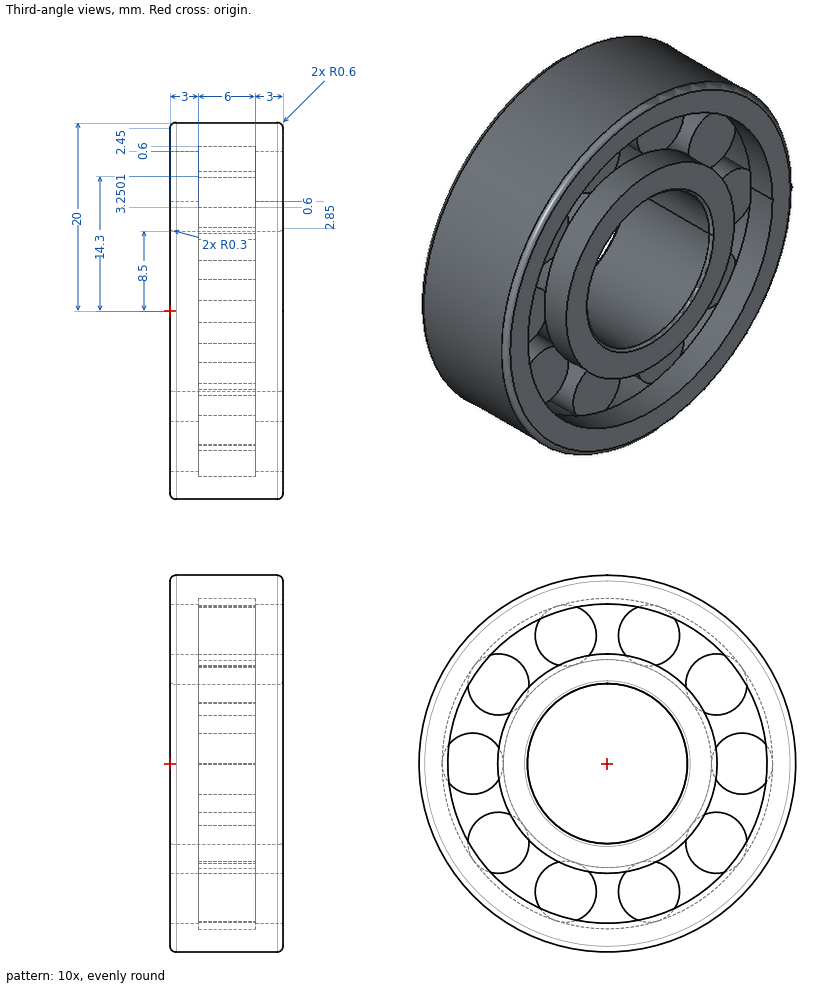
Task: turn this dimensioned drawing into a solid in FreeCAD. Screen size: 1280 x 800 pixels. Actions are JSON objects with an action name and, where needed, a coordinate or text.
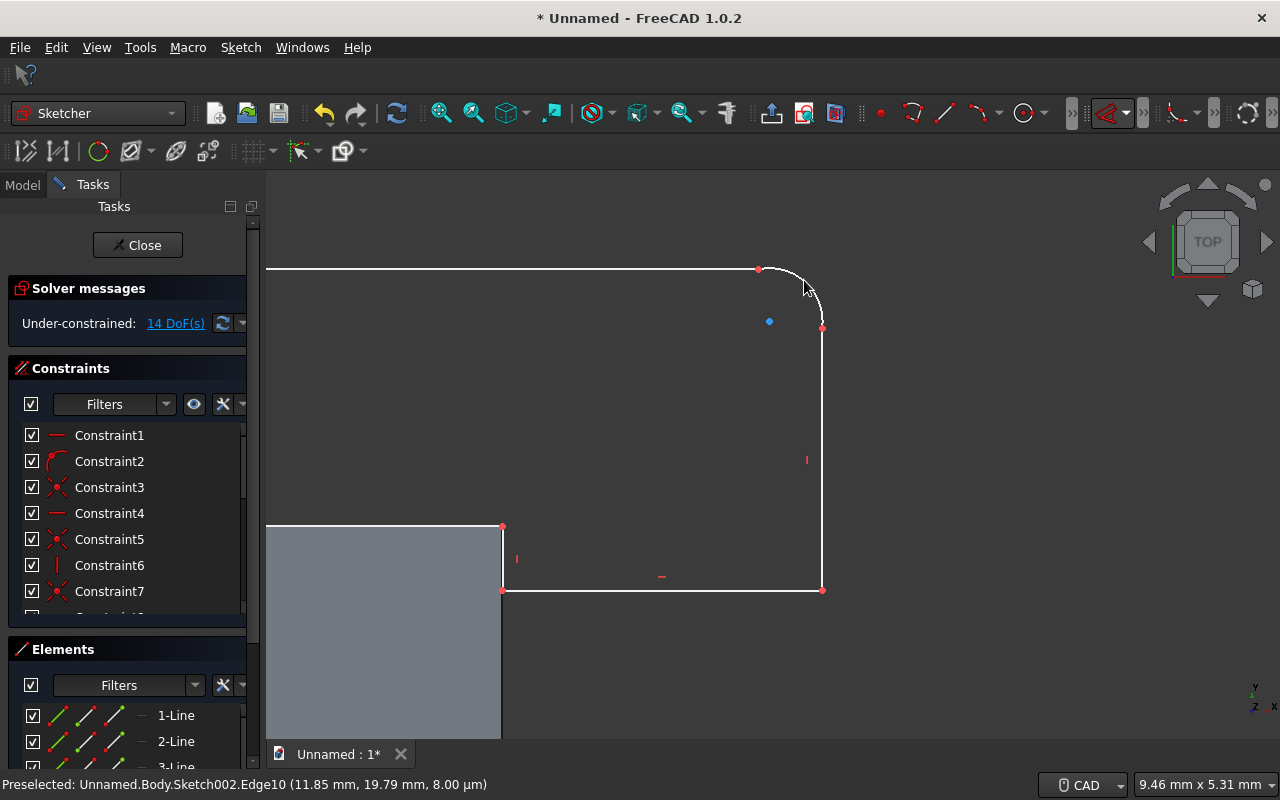
{"action": "scroll", "coordinate": [808, 280], "scroll_direction": "down", "scroll_amount": 9}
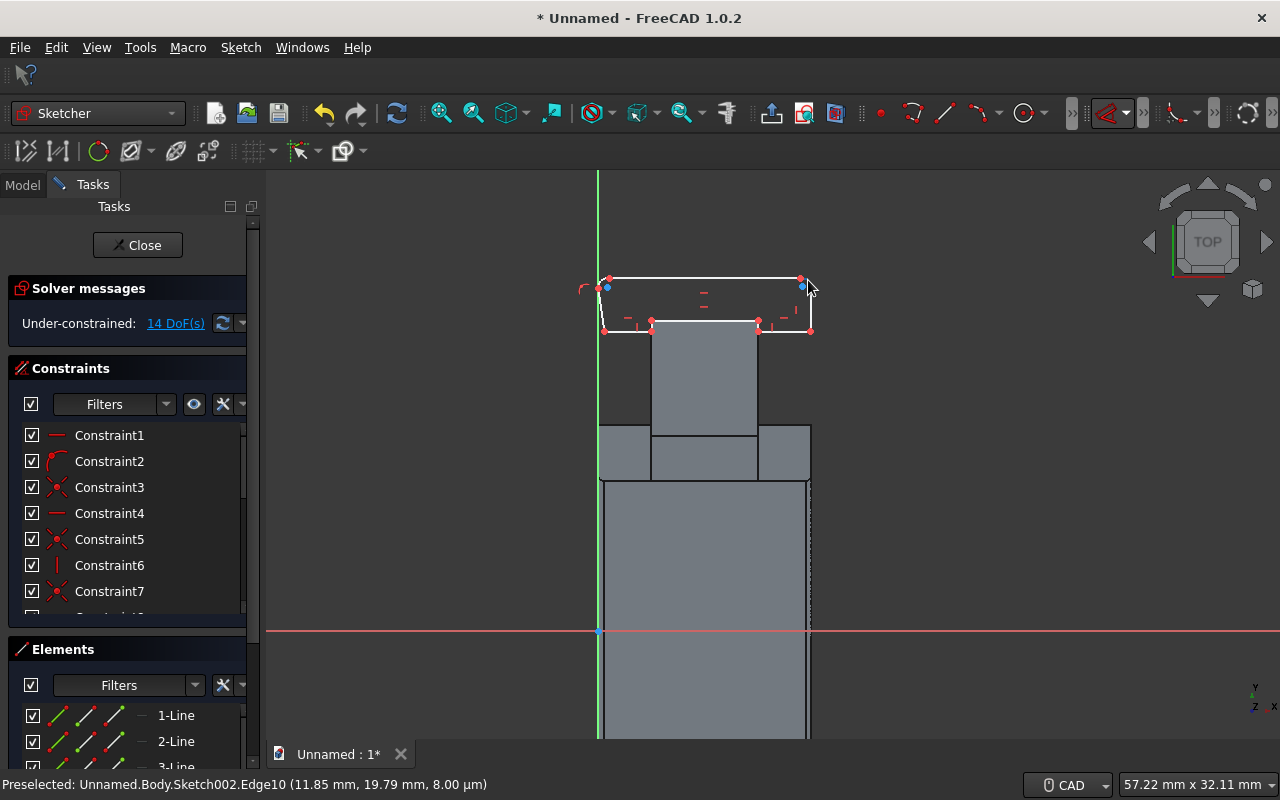
{"action": "left_click", "coordinate": [743, 278]}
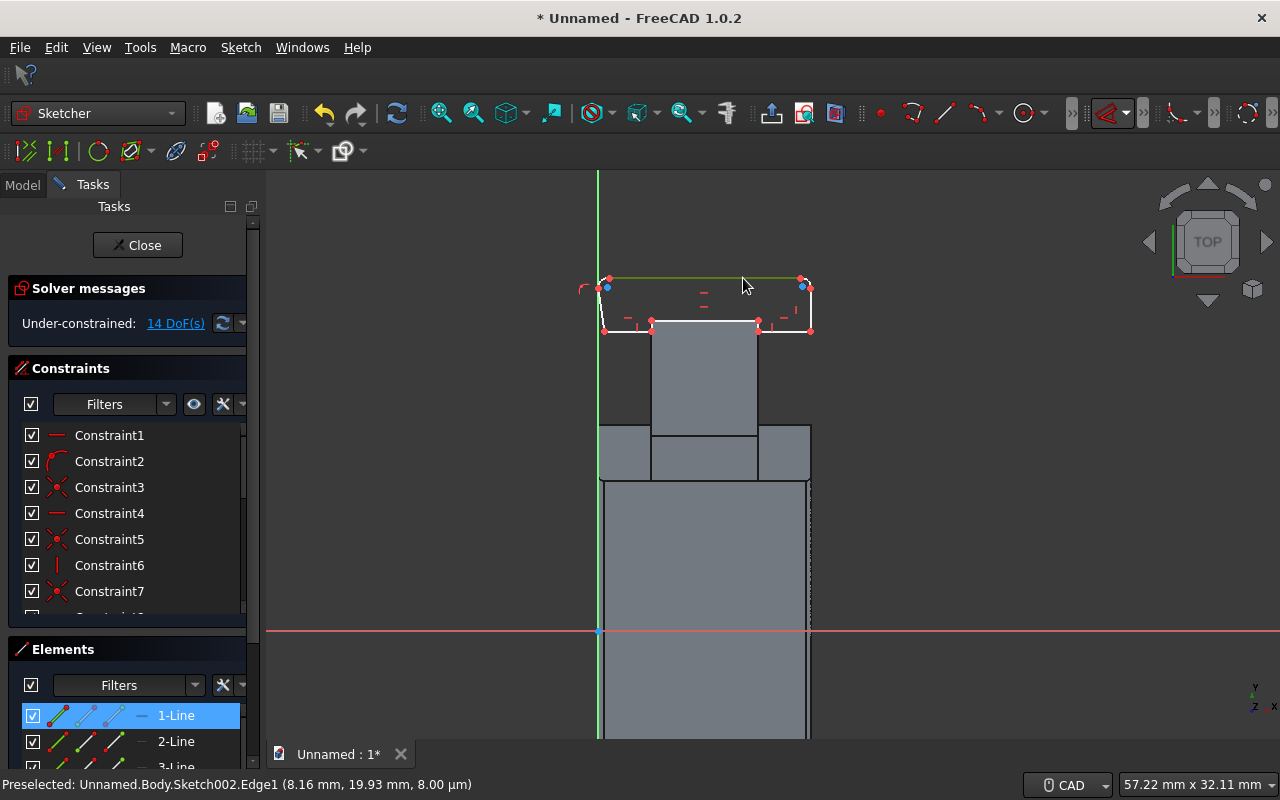
{"action": "scroll", "coordinate": [601, 281], "scroll_direction": "up", "scroll_amount": 3}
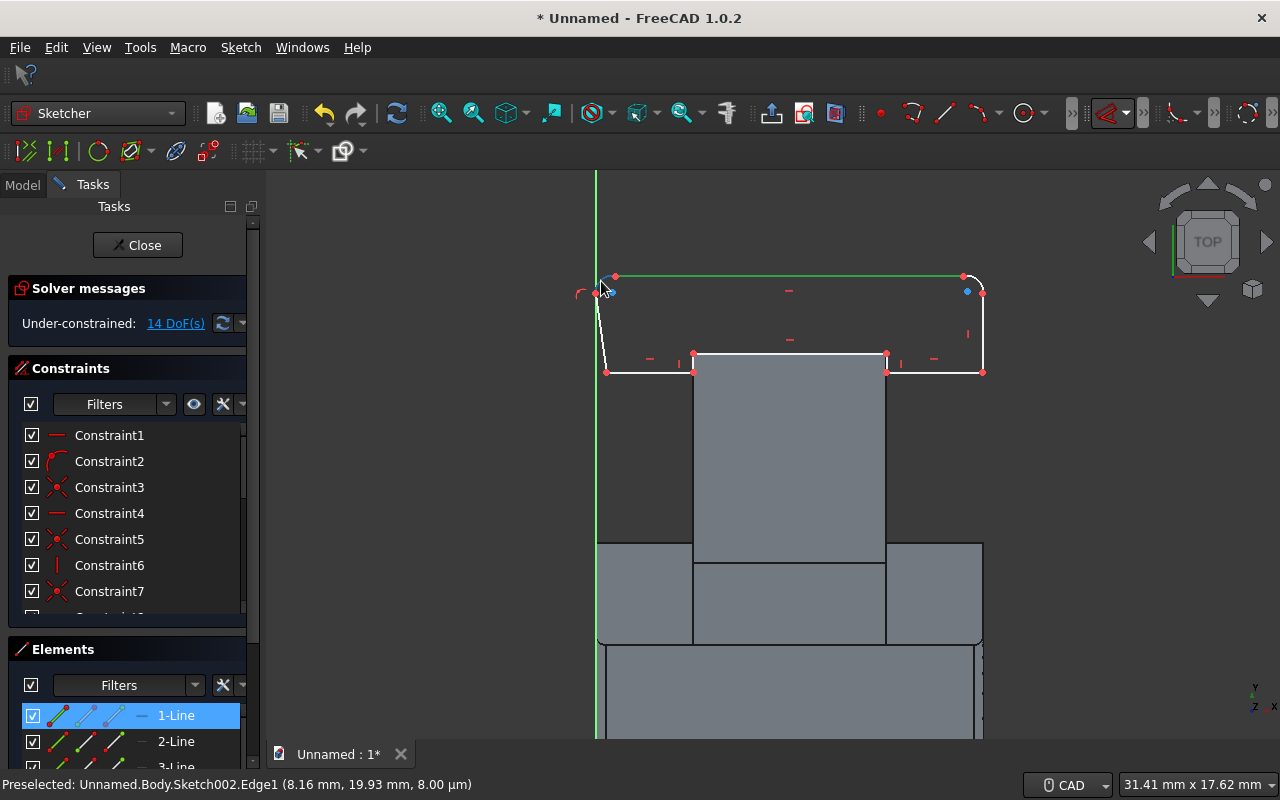
{"action": "left_click", "coordinate": [601, 280]}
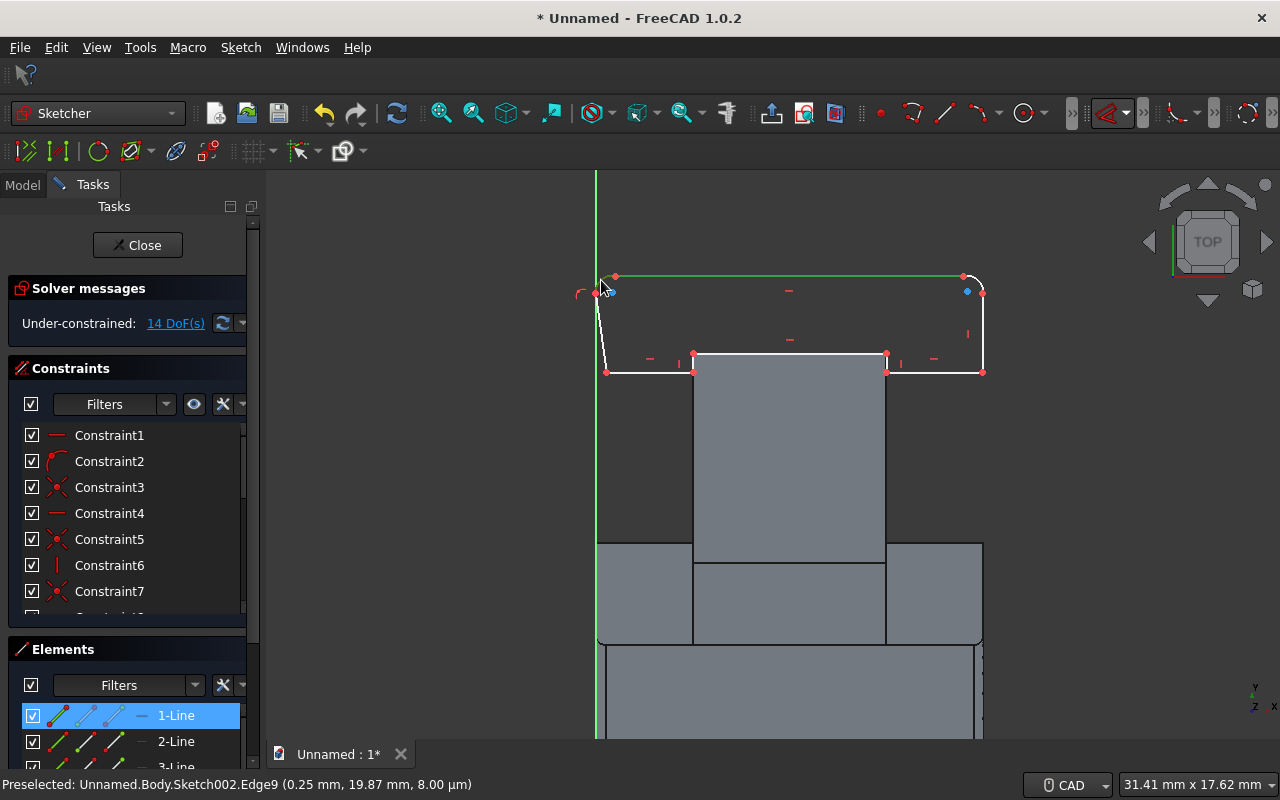
{"action": "key", "text": "t"}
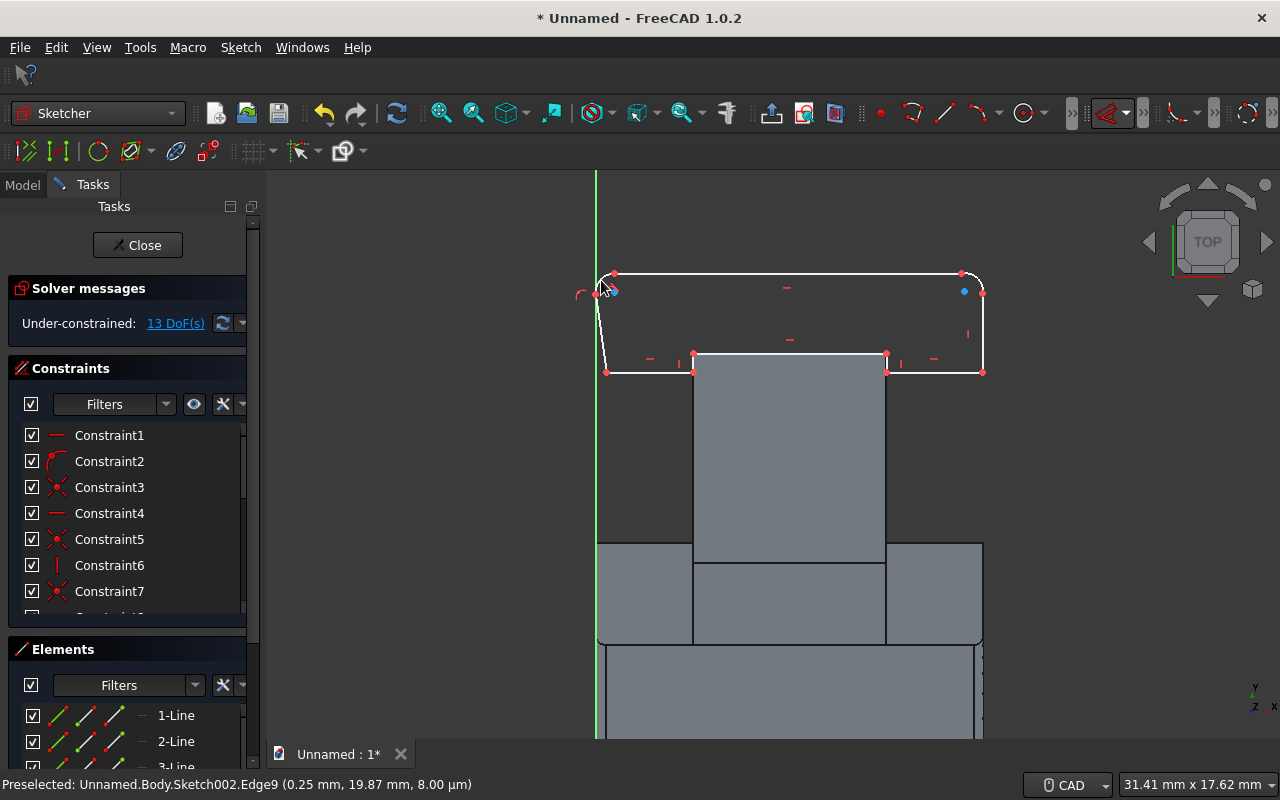
{"action": "left_click", "coordinate": [857, 274]}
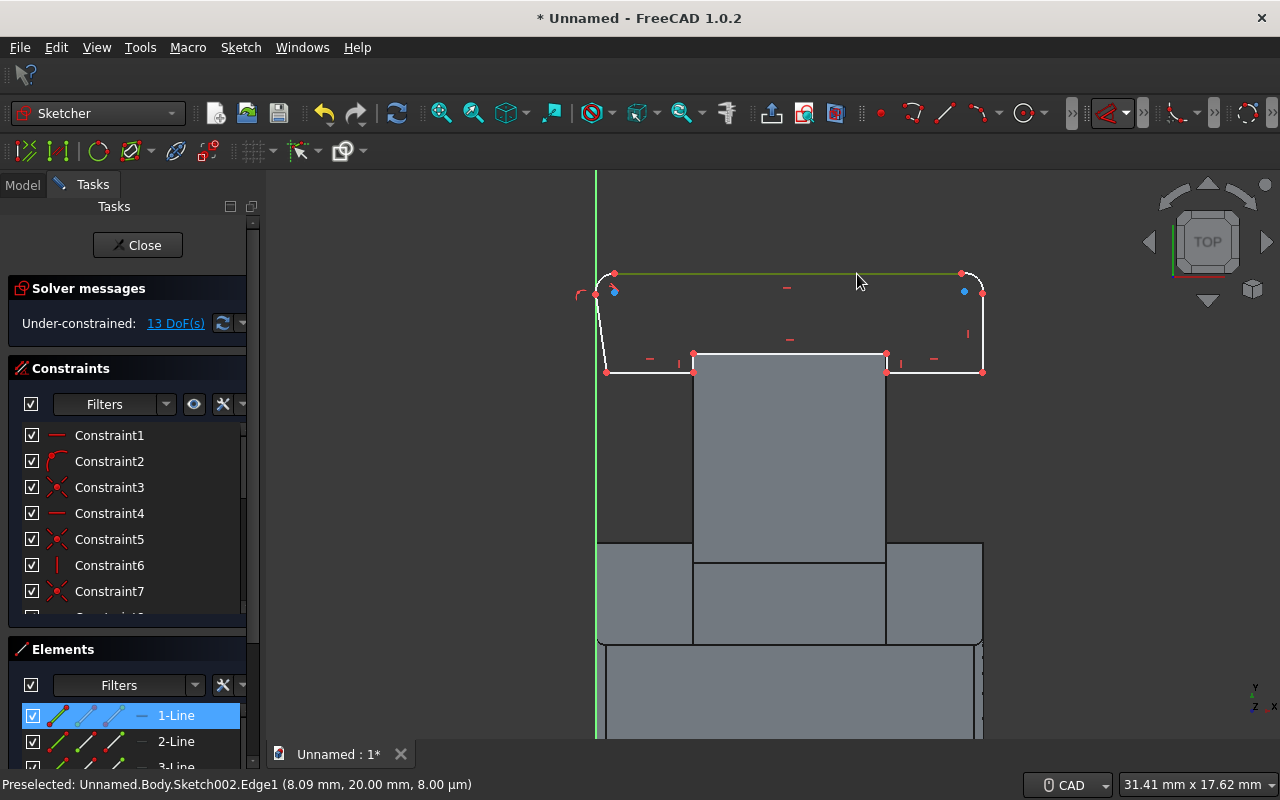
{"action": "scroll", "coordinate": [981, 284], "scroll_direction": "up", "scroll_amount": 2}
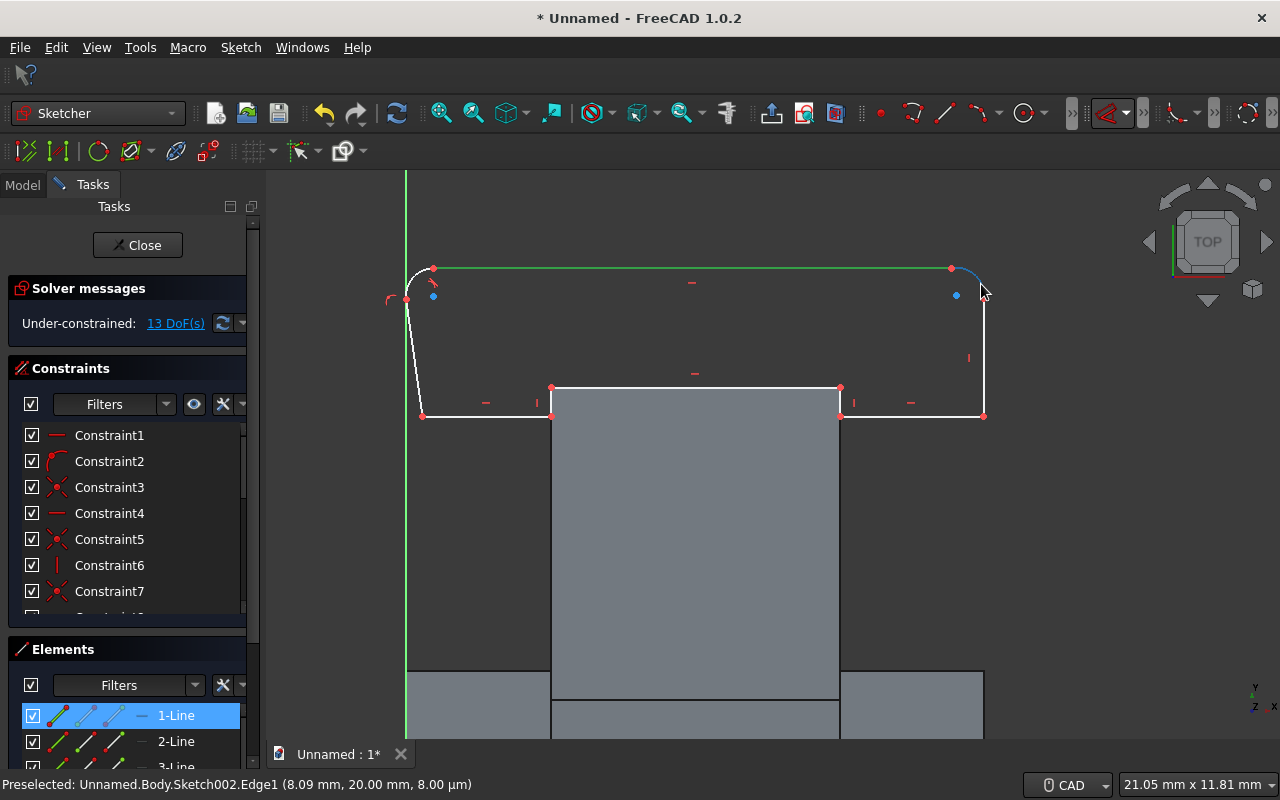
{"action": "left_click", "coordinate": [981, 283]}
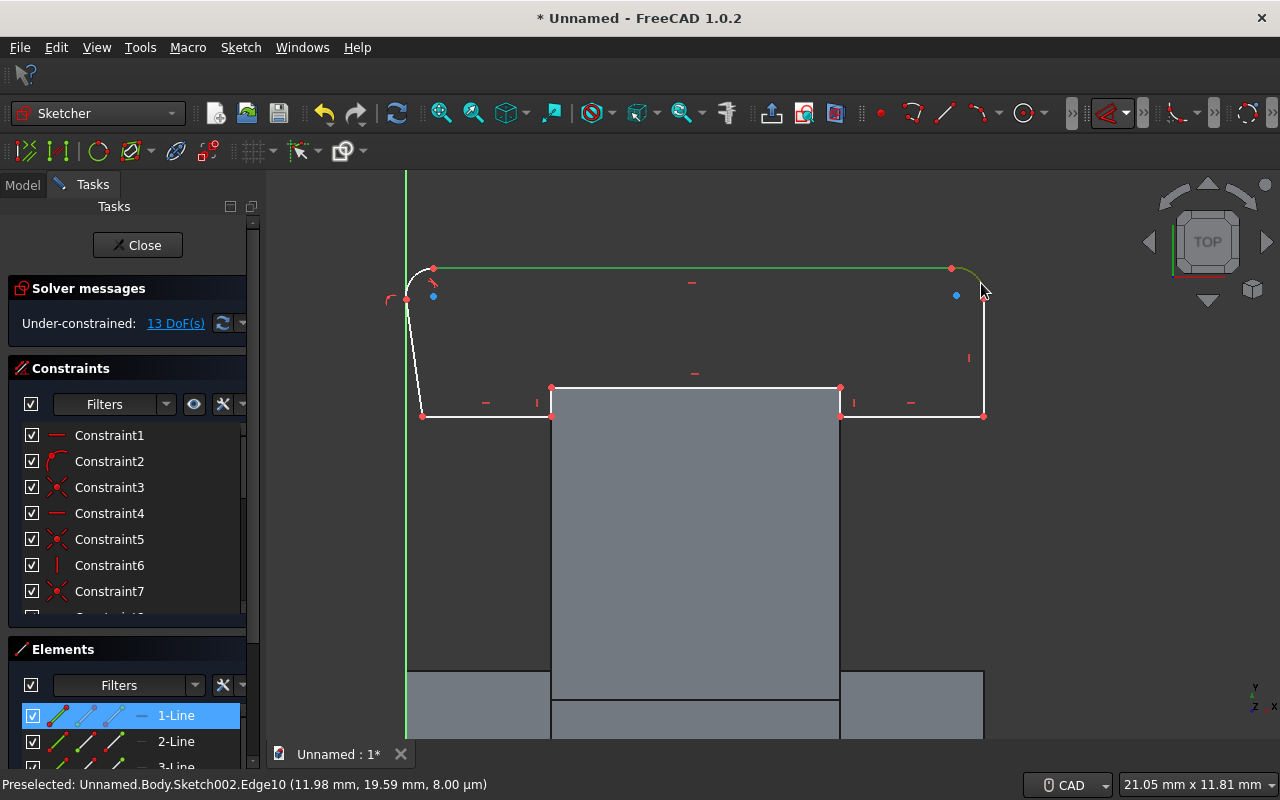
{"action": "key", "text": "t"}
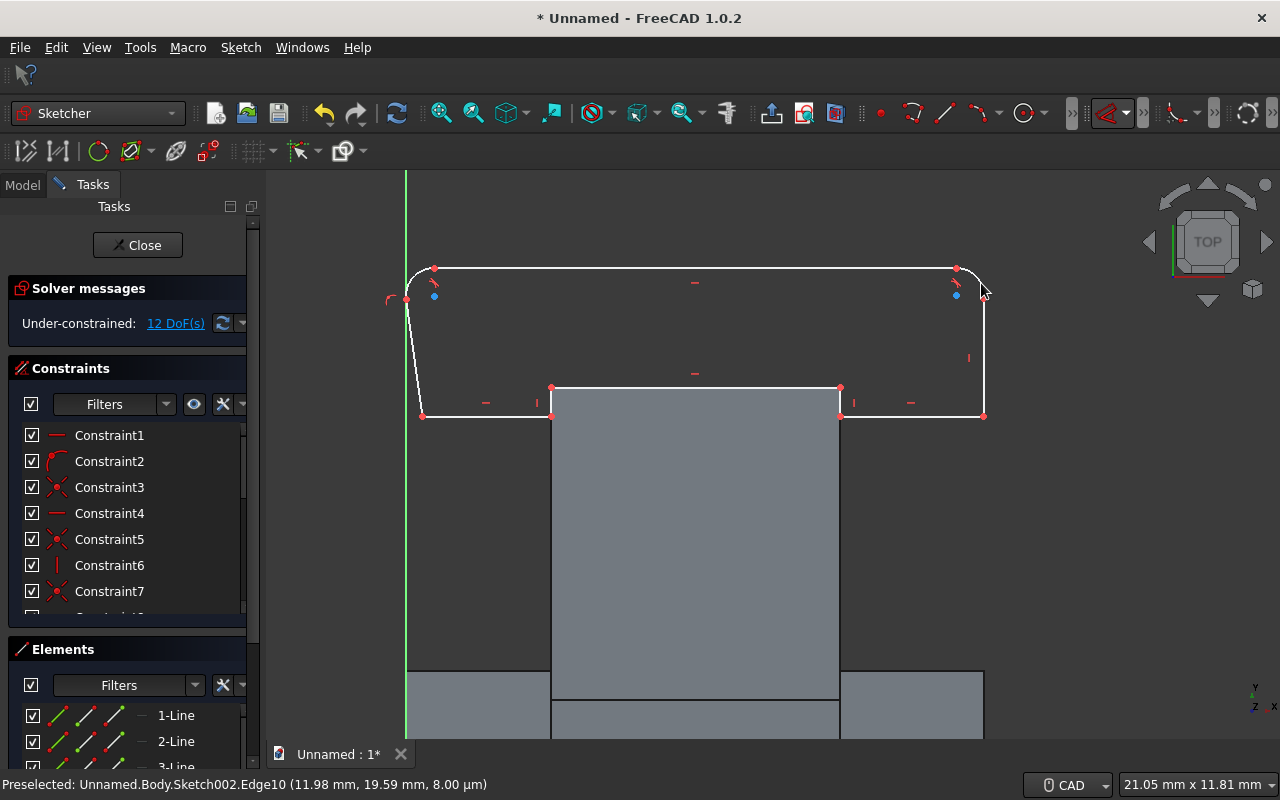
{"action": "left_click", "coordinate": [418, 381]}